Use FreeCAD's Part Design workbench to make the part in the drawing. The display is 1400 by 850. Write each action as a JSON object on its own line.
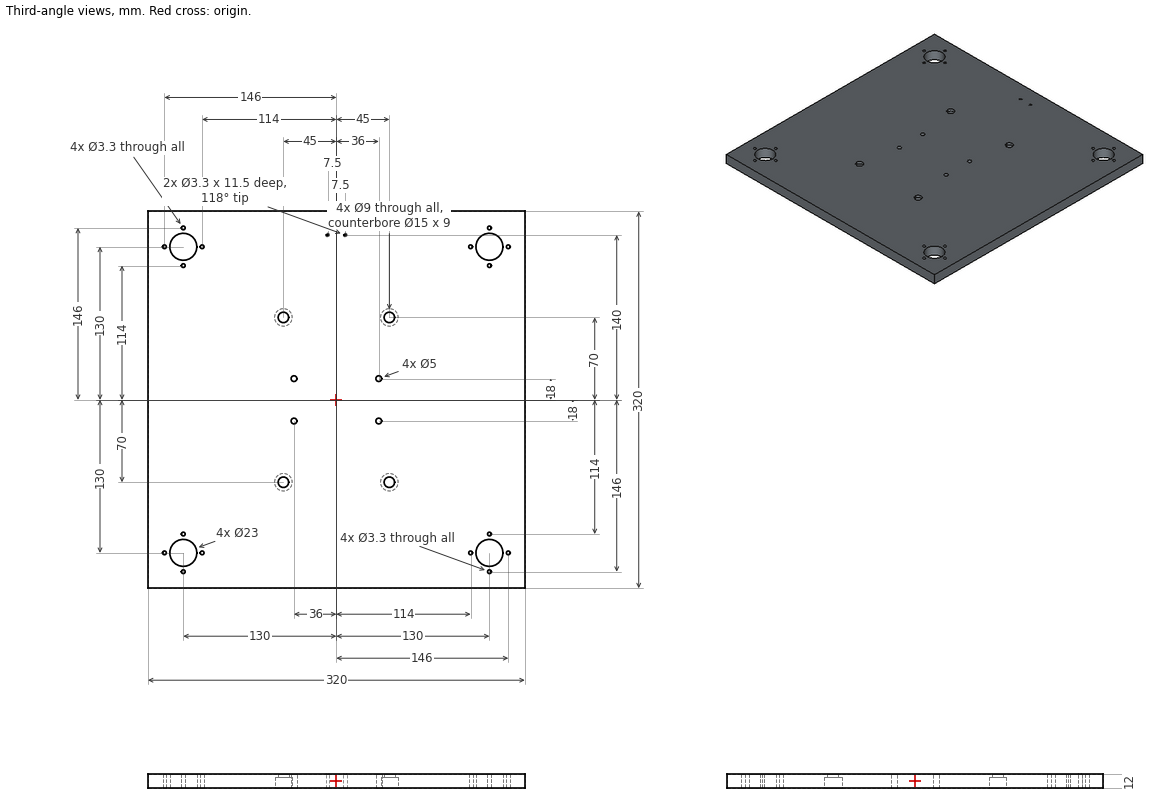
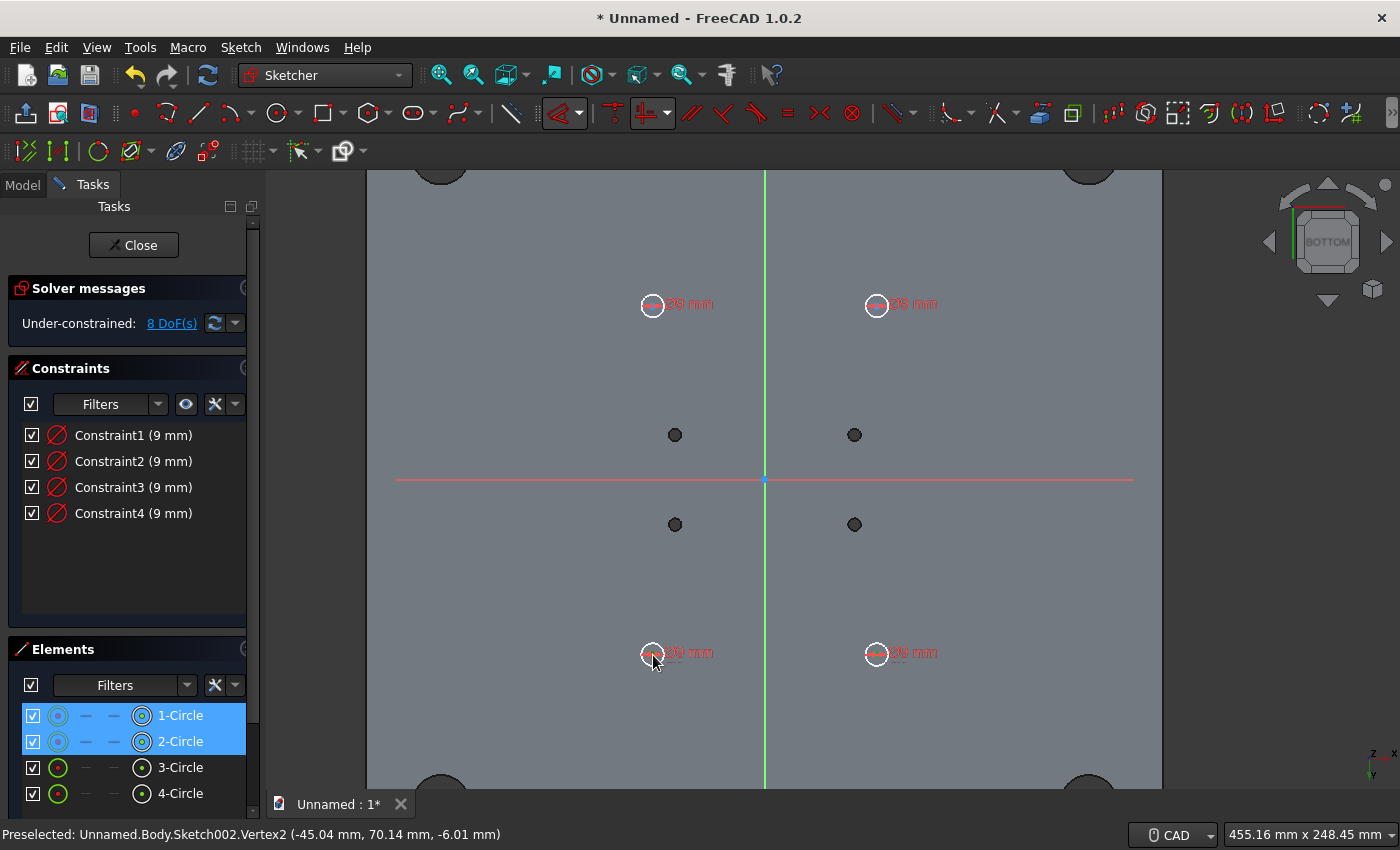
{"action": "key", "text": "h"}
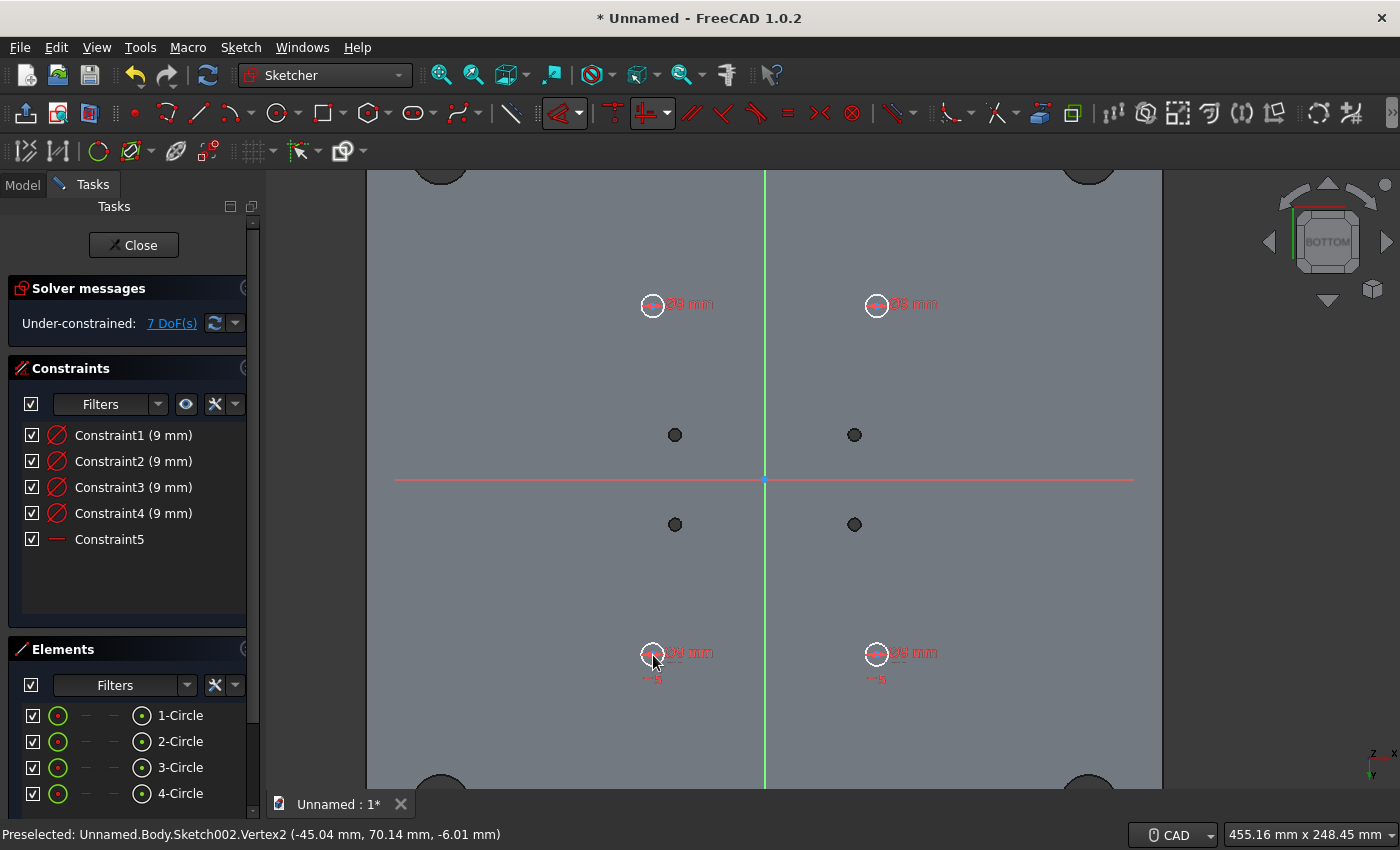
{"action": "left_click", "coordinate": [653, 655]}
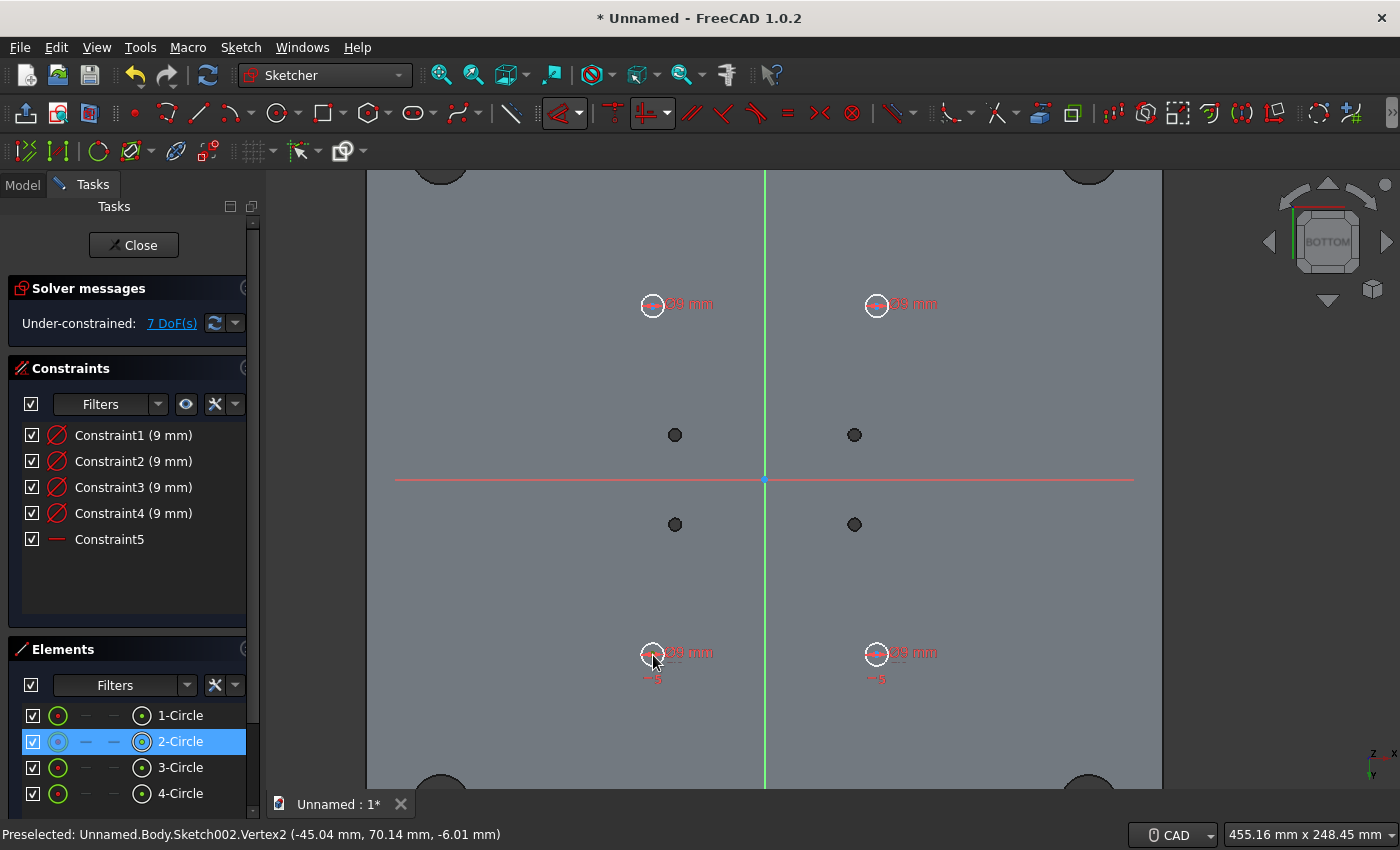
{"action": "left_click", "coordinate": [653, 306]}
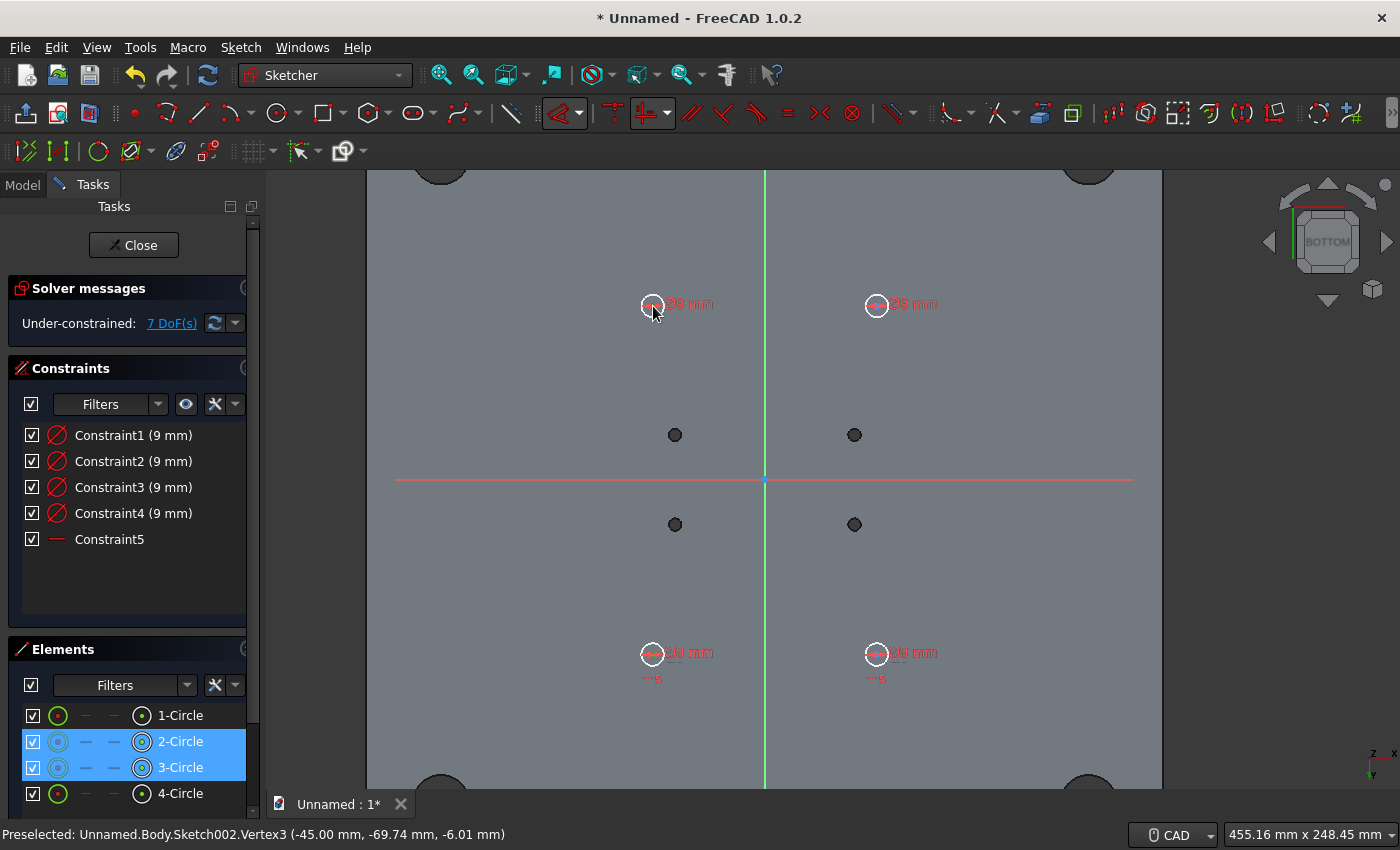
{"action": "key", "text": "v"}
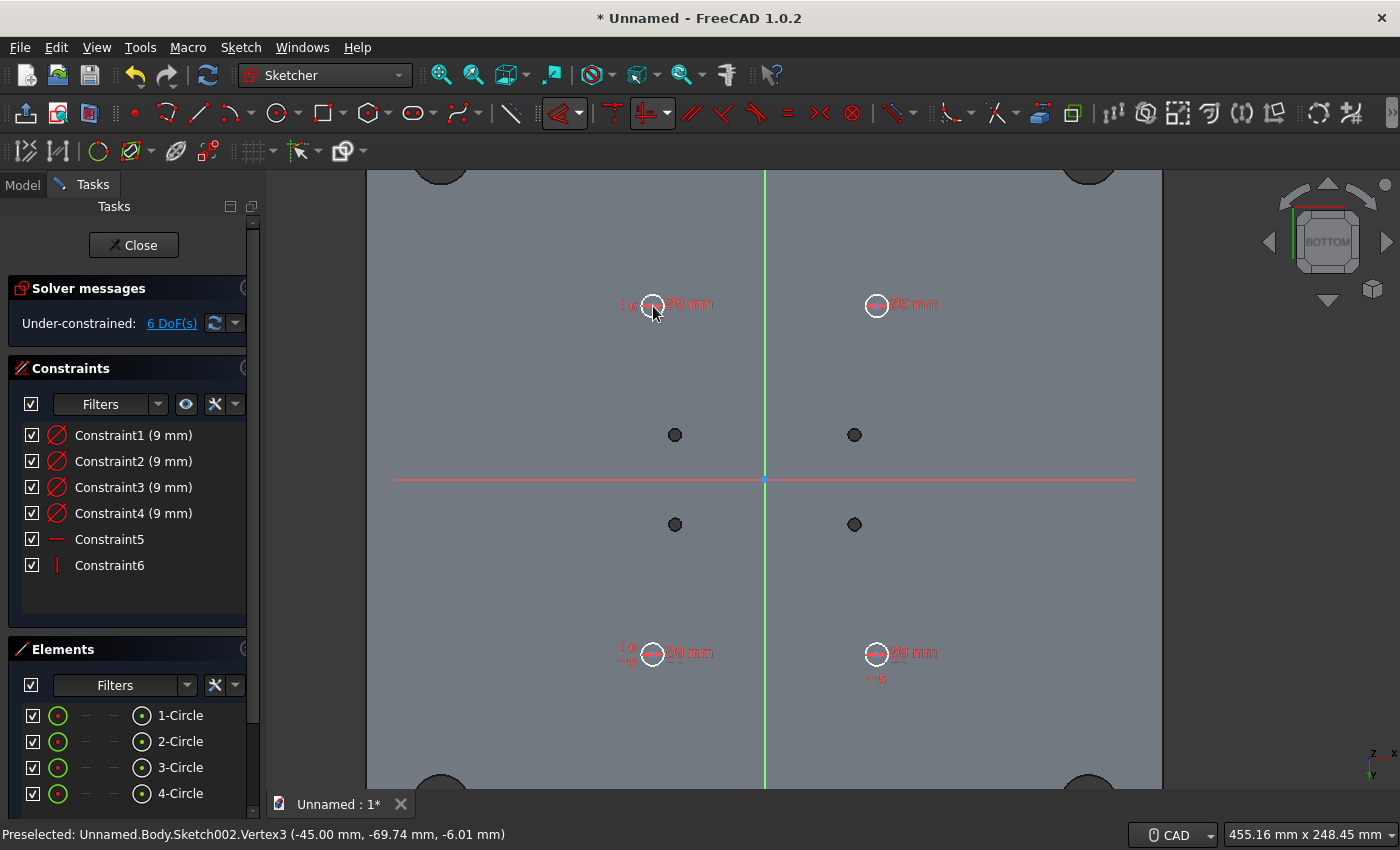
{"action": "left_click", "coordinate": [877, 655]}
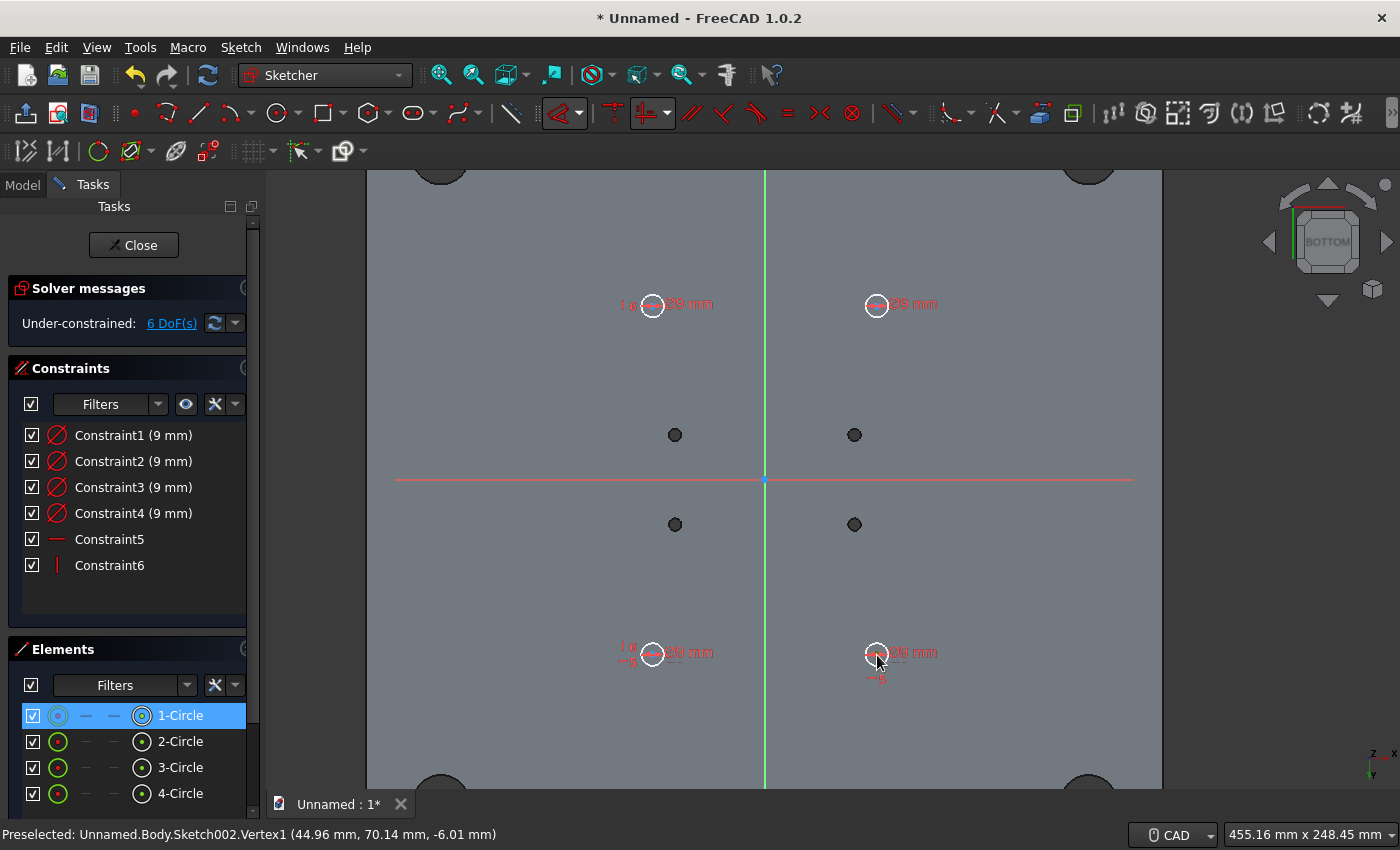
{"action": "left_click", "coordinate": [877, 306]}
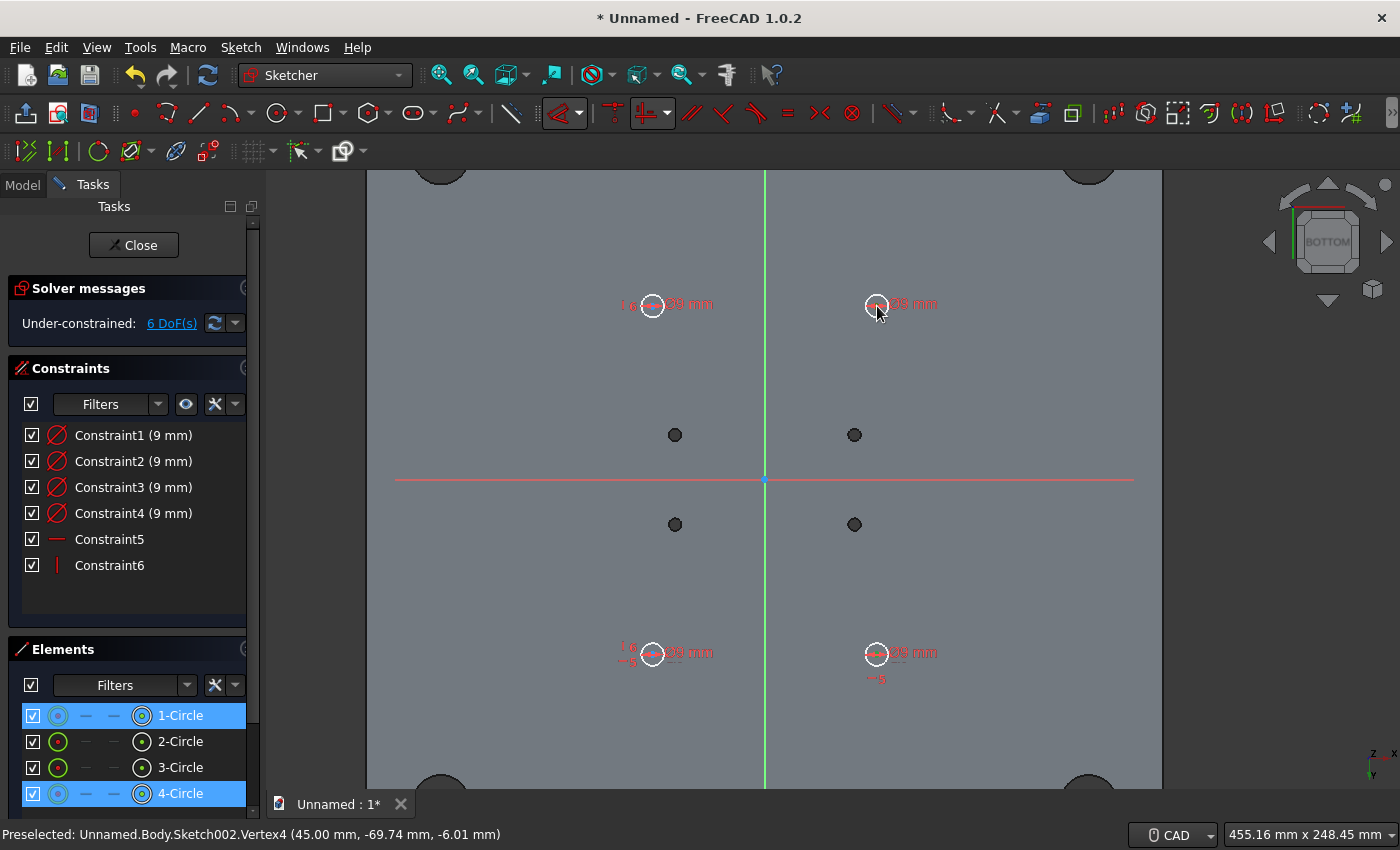
{"action": "left_click", "coordinate": [670, 114]}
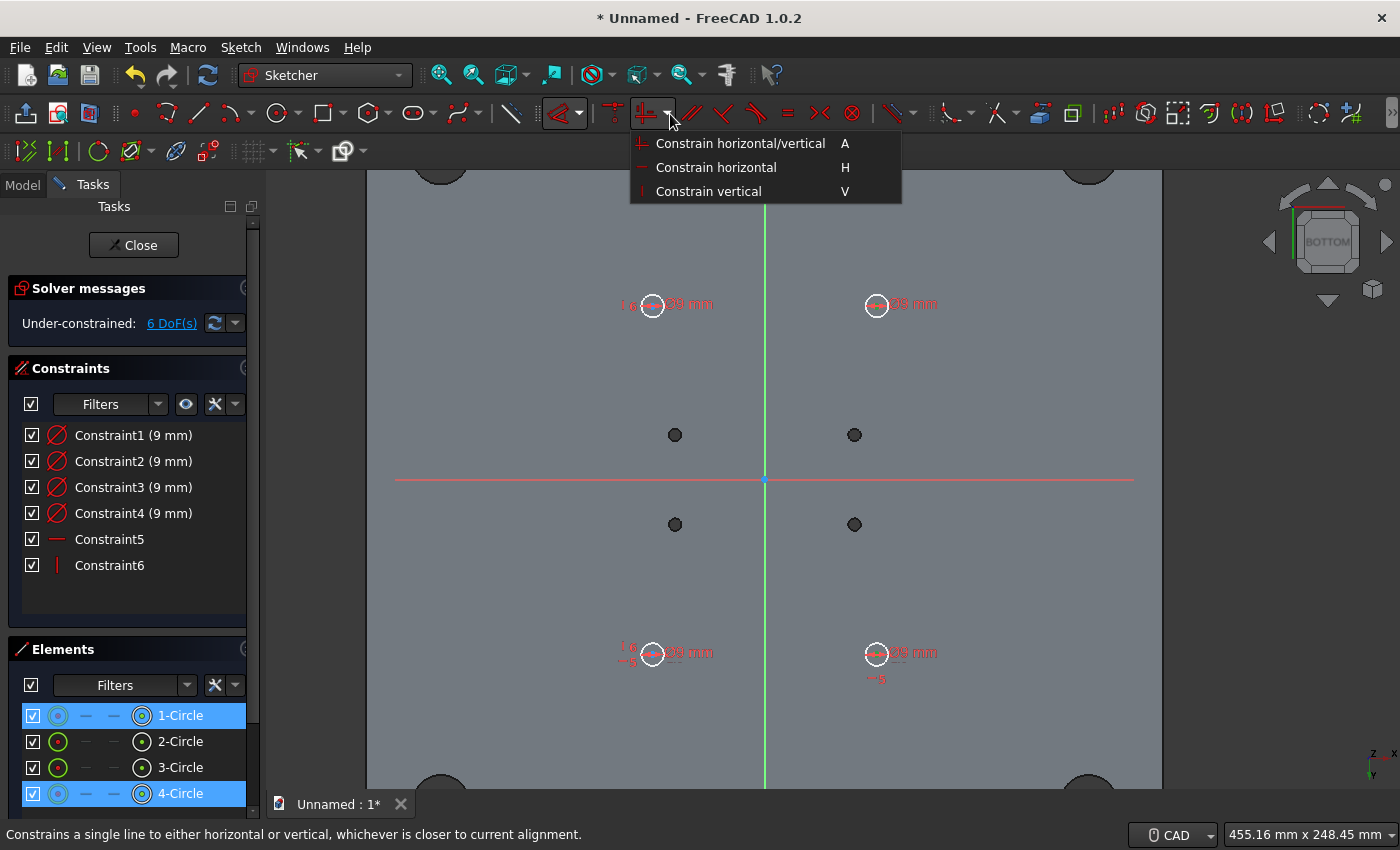
{"action": "left_click", "coordinate": [766, 191]}